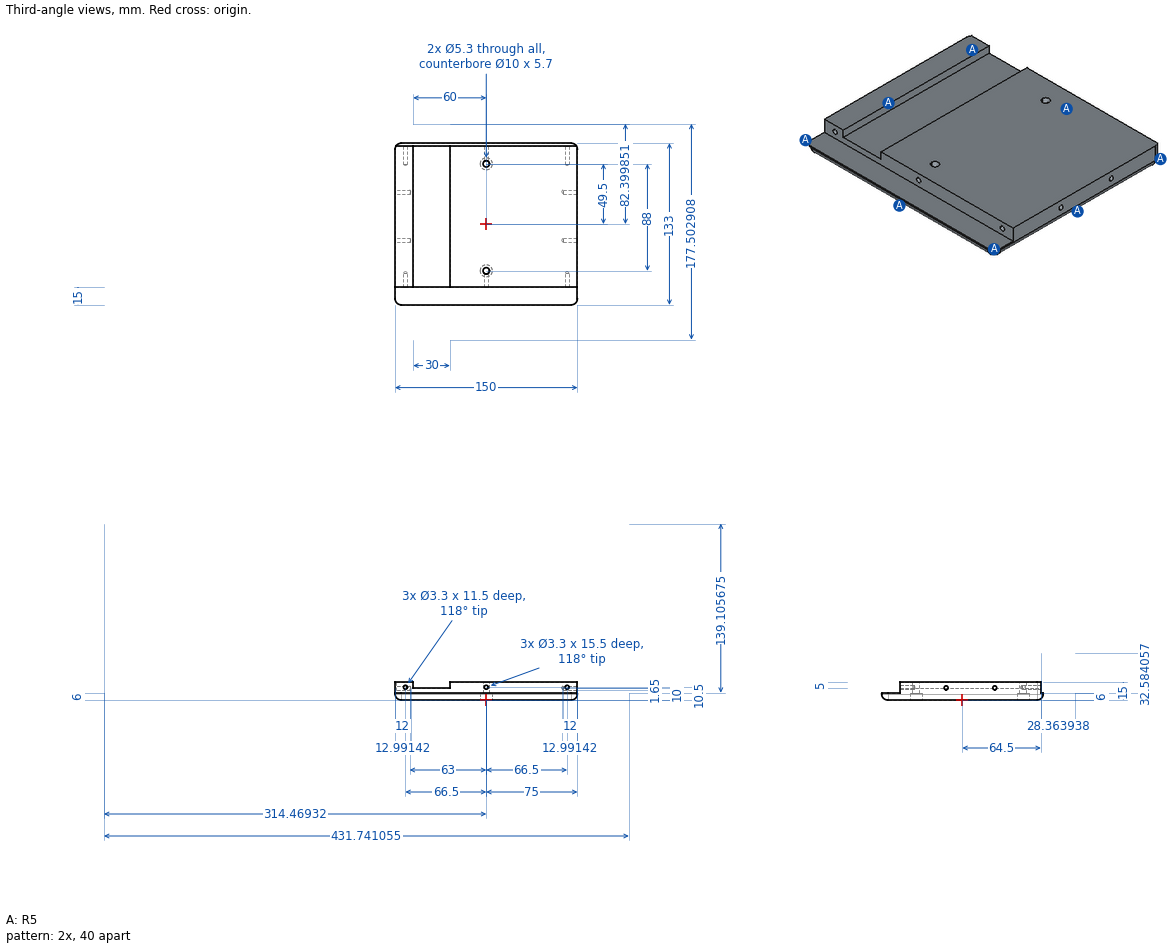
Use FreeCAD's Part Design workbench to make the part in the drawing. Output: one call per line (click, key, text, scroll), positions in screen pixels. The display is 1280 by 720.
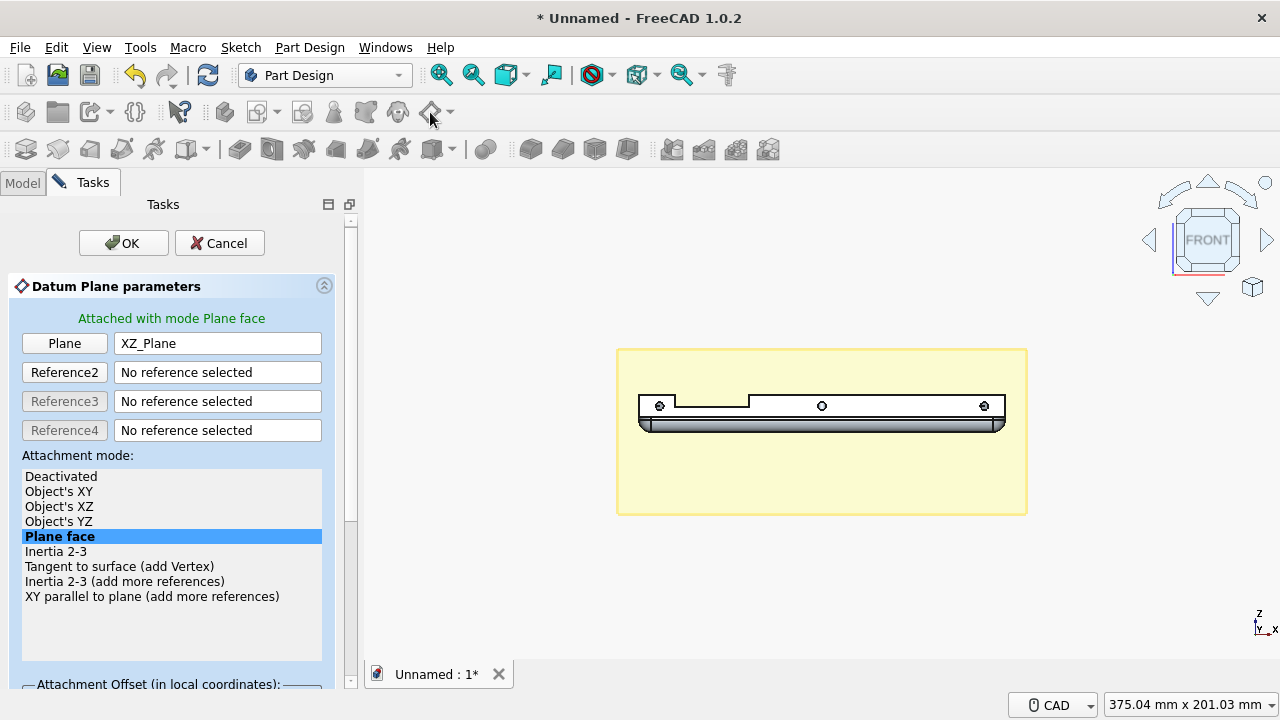
scroll(351, 451, down, 3)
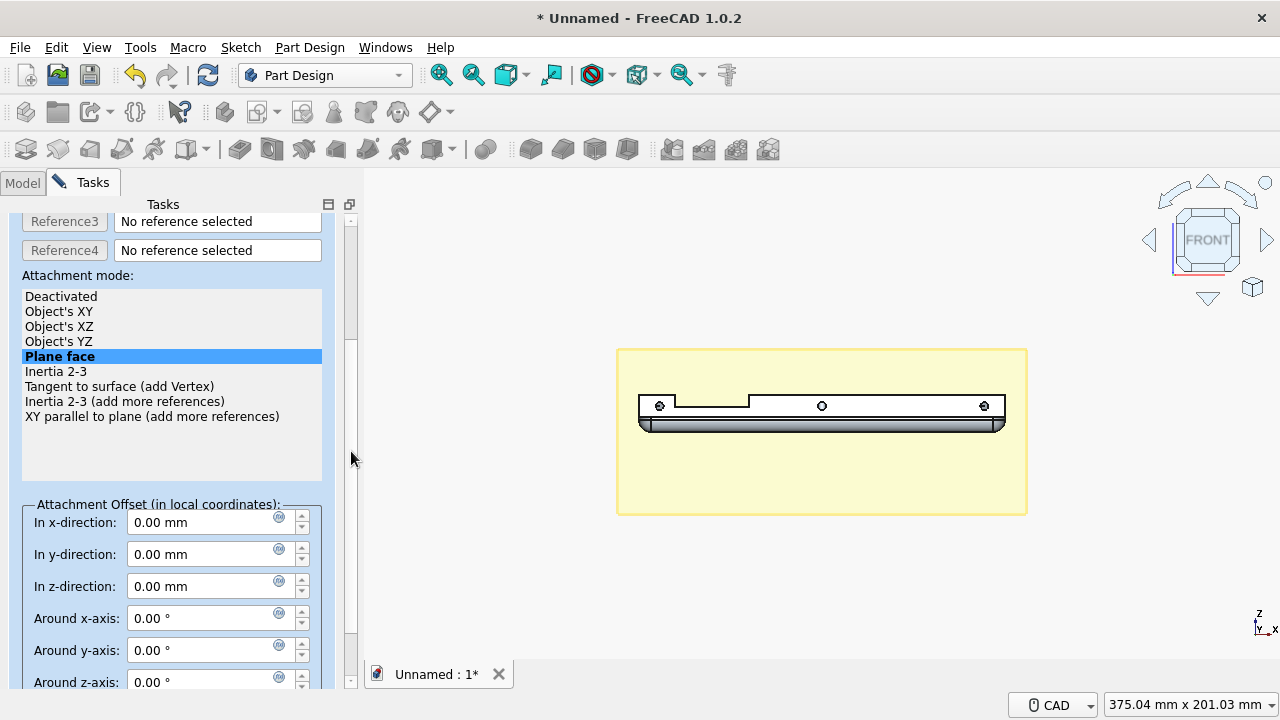
triple_click(210, 586)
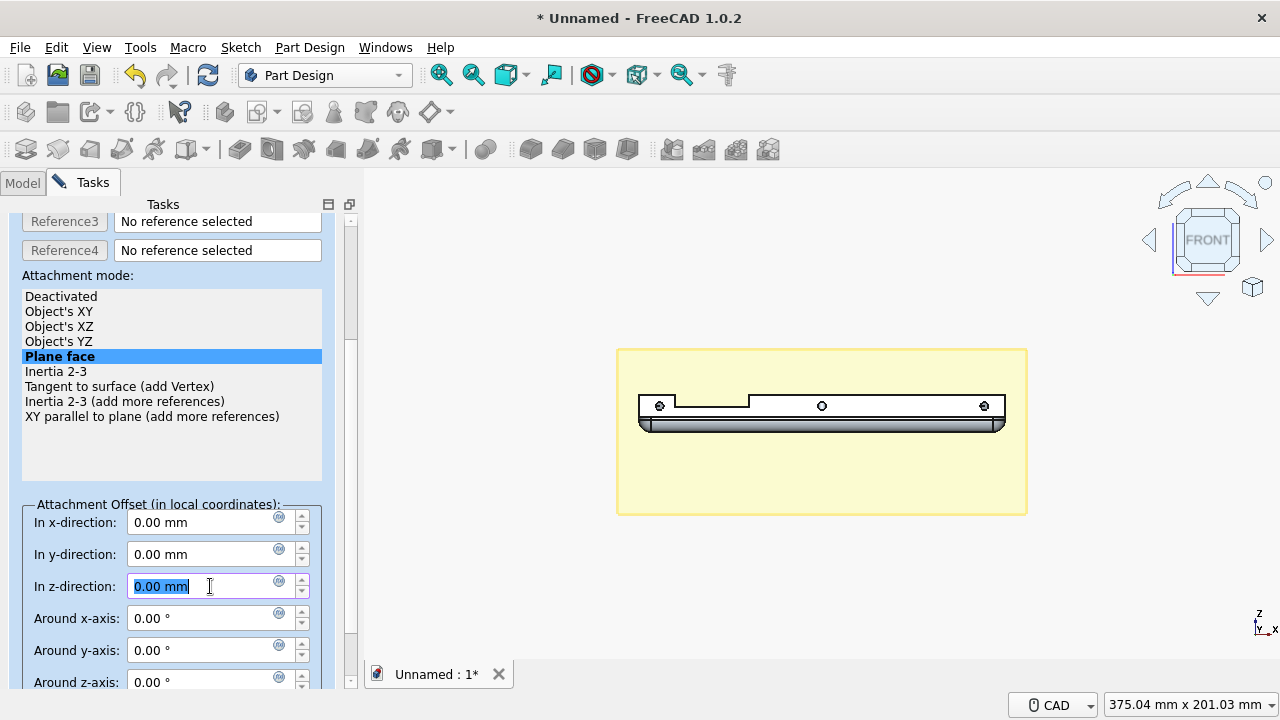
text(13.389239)
key(Tab)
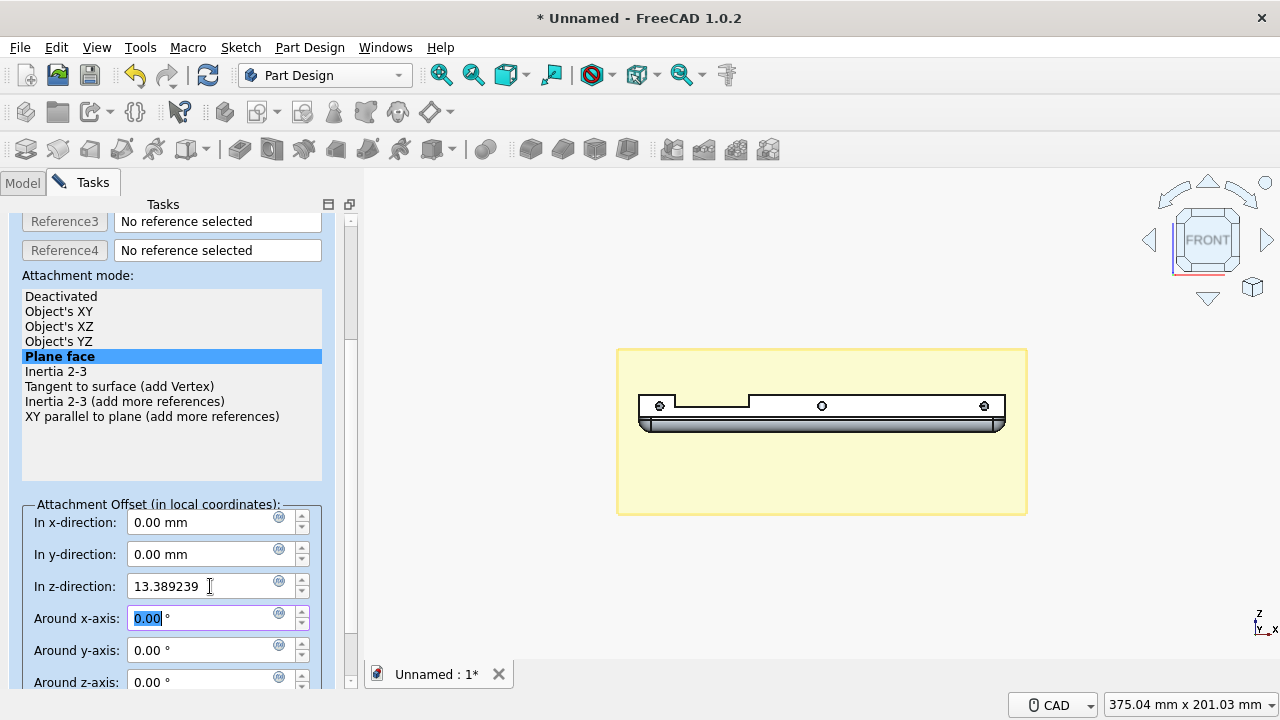
scroll(351, 451, up, 4)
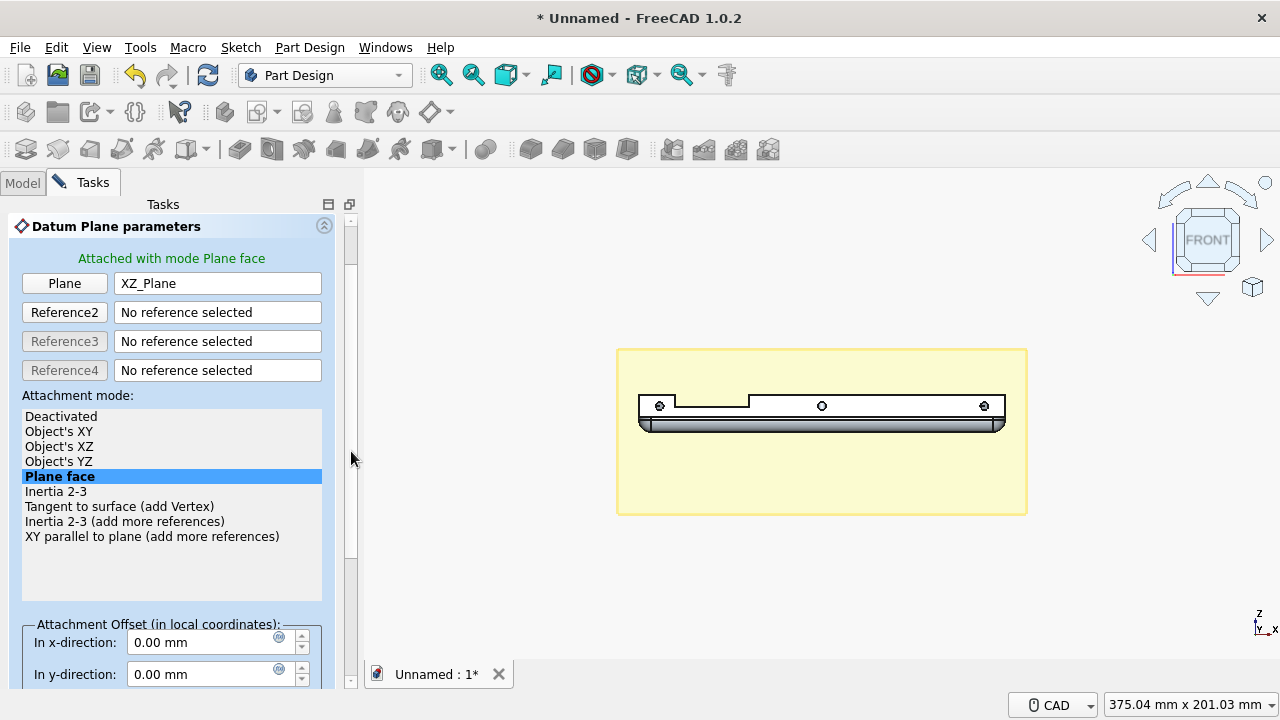
click(124, 243)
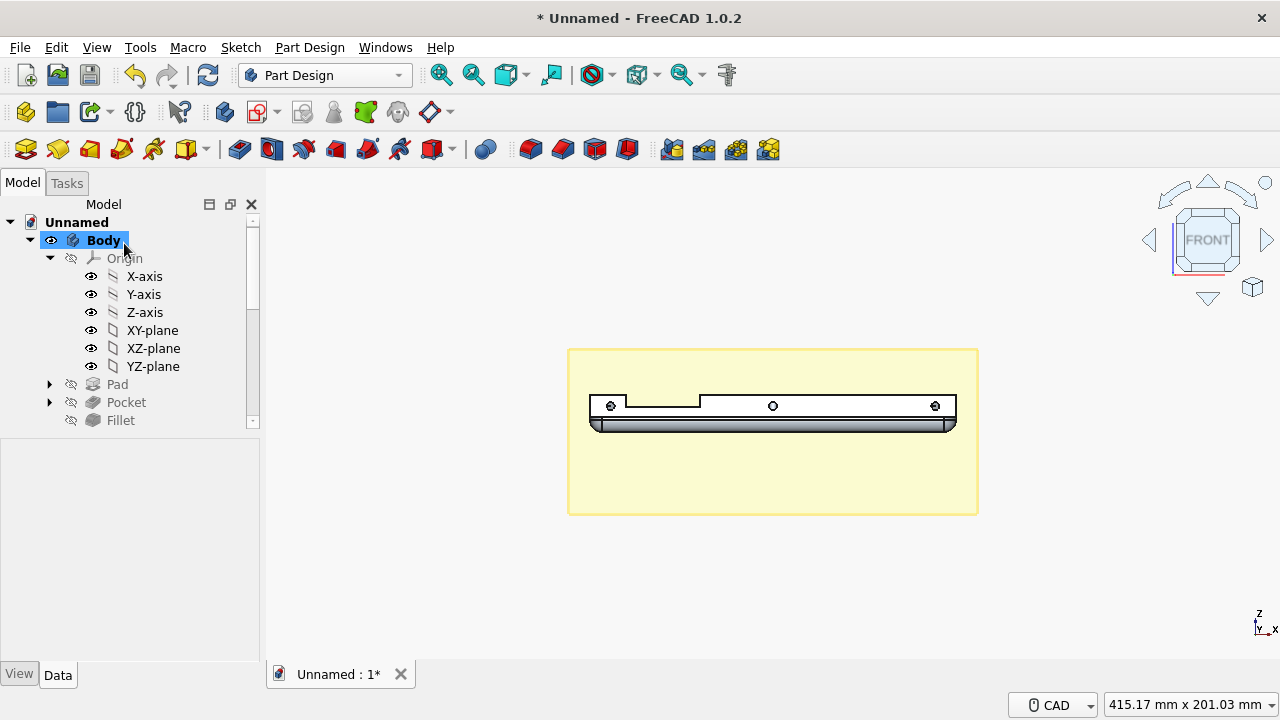
scroll(100, 326, down, 3)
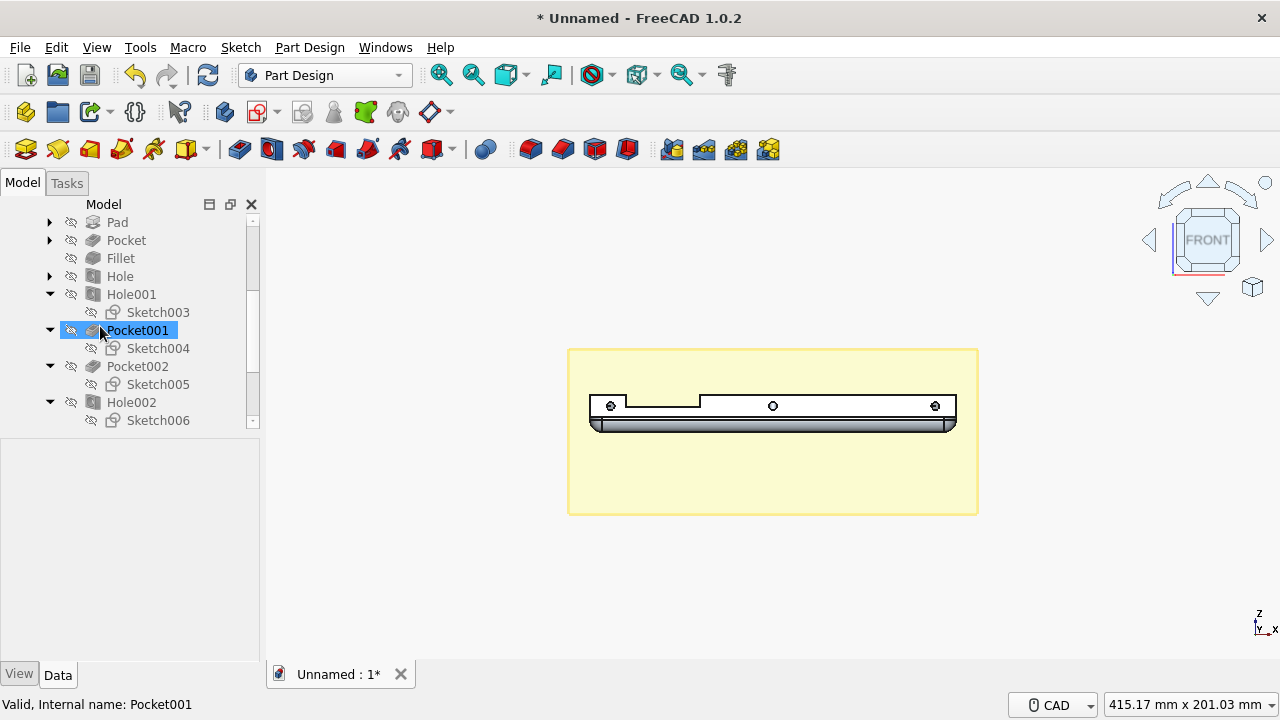
scroll(140, 326, up, 15)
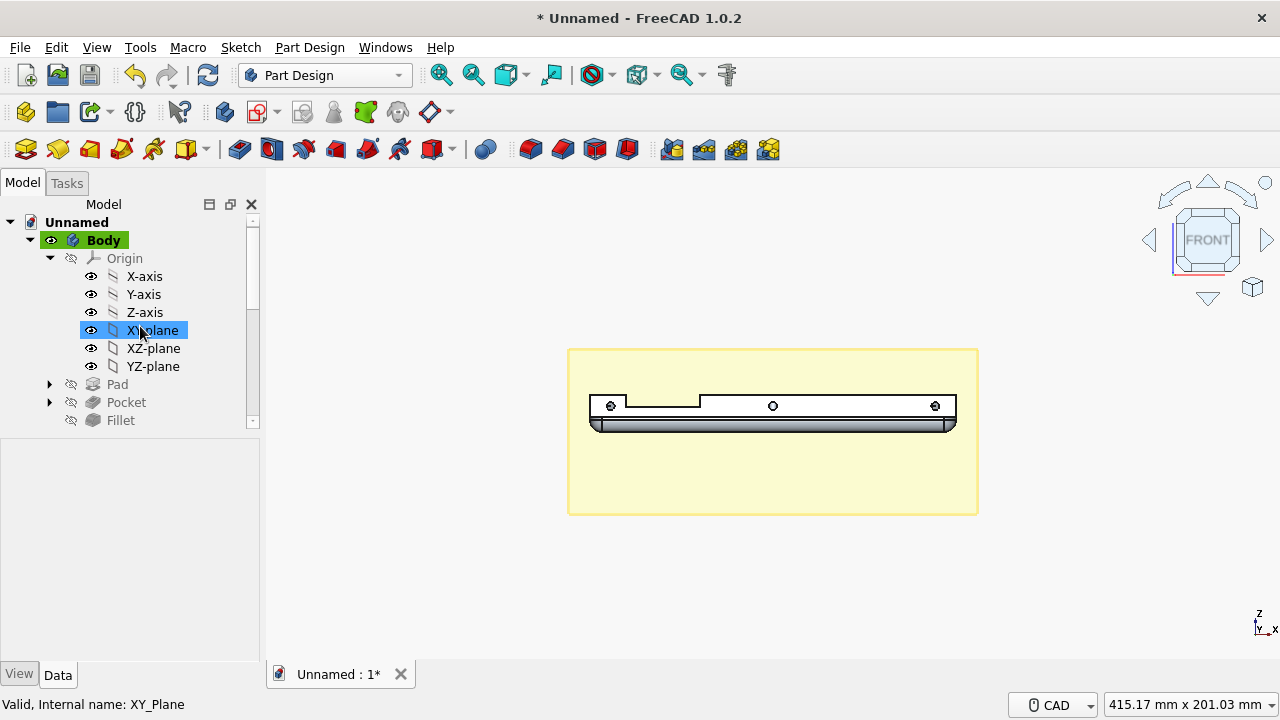
scroll(100, 326, down, 6)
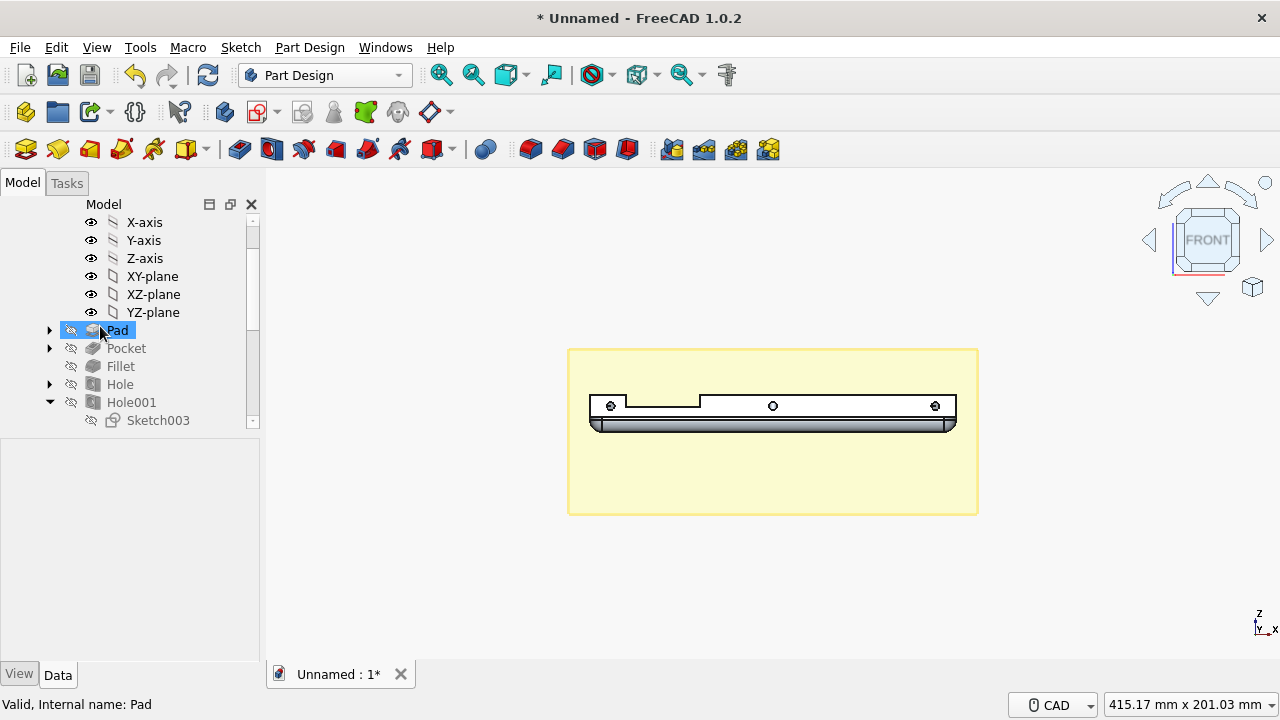
click(116, 420)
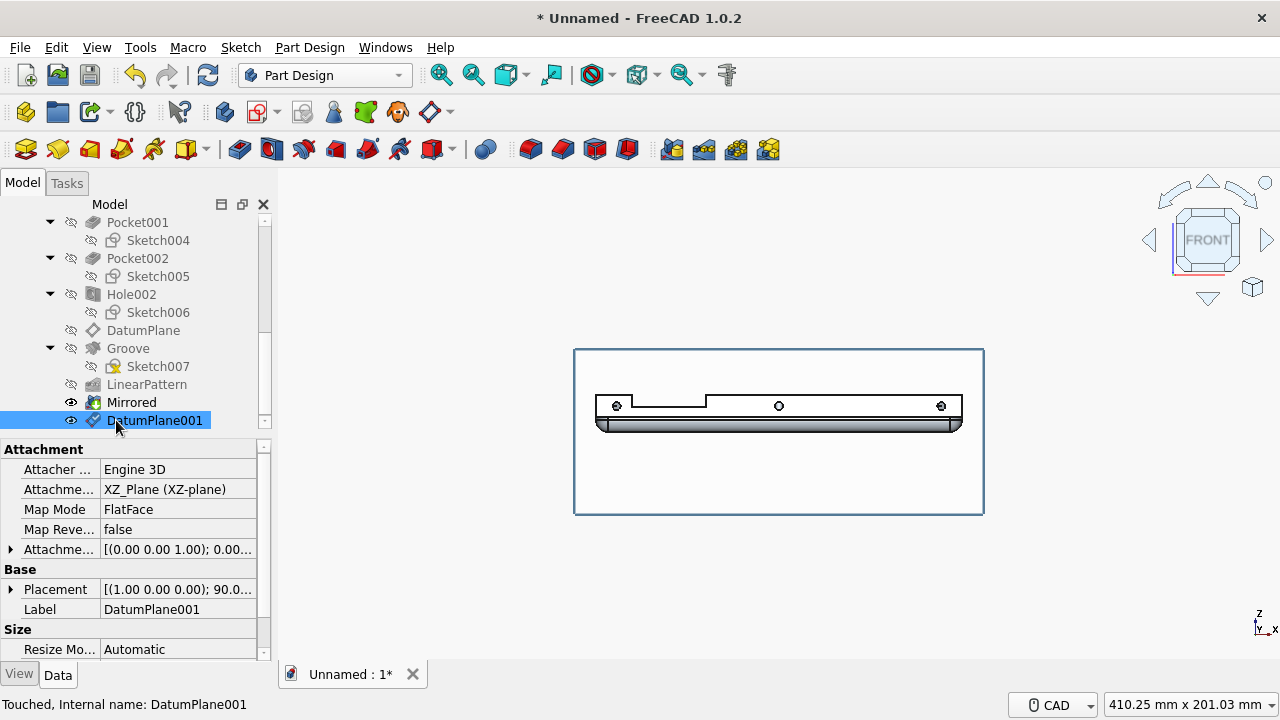
click(258, 112)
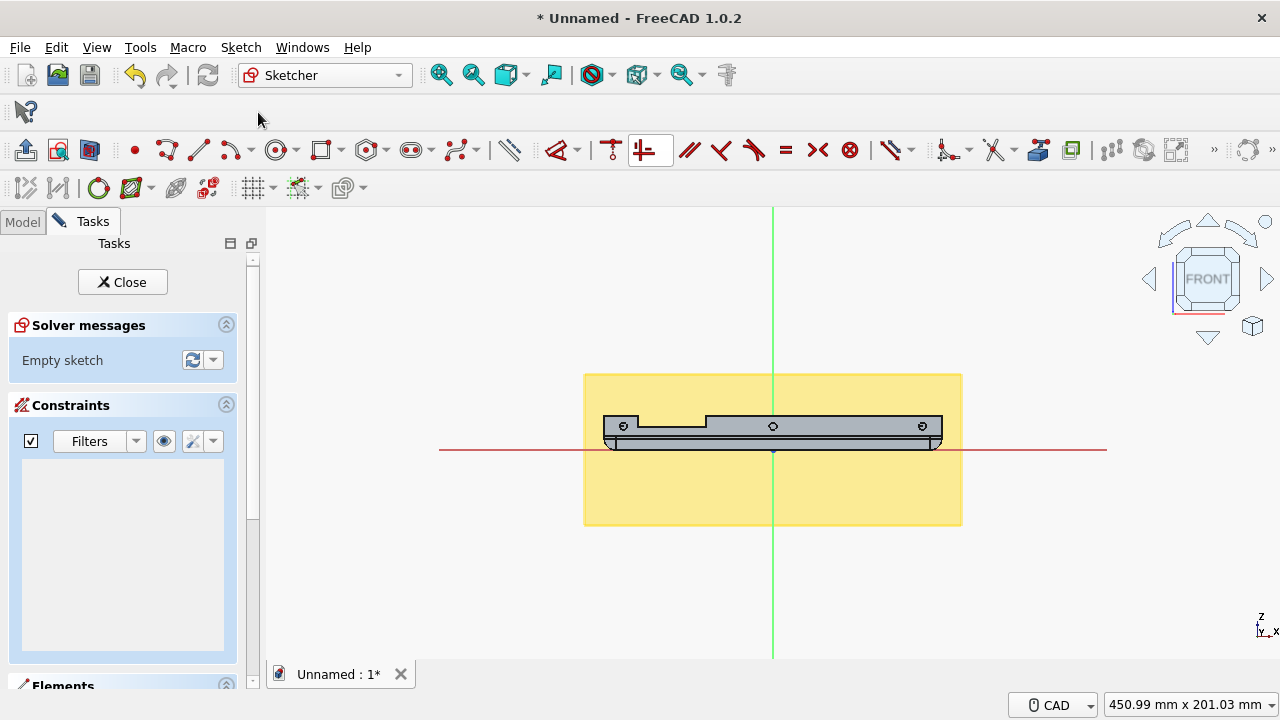
click(90, 150)